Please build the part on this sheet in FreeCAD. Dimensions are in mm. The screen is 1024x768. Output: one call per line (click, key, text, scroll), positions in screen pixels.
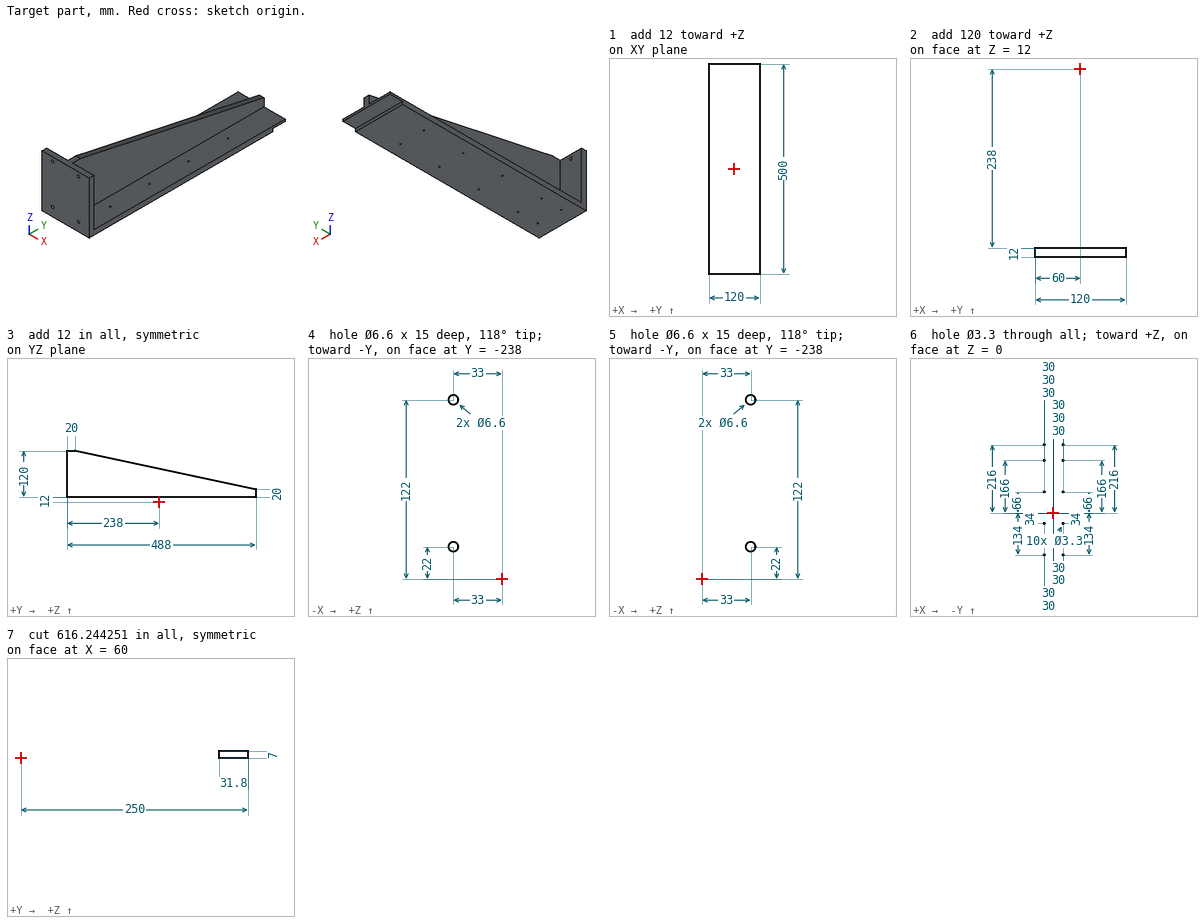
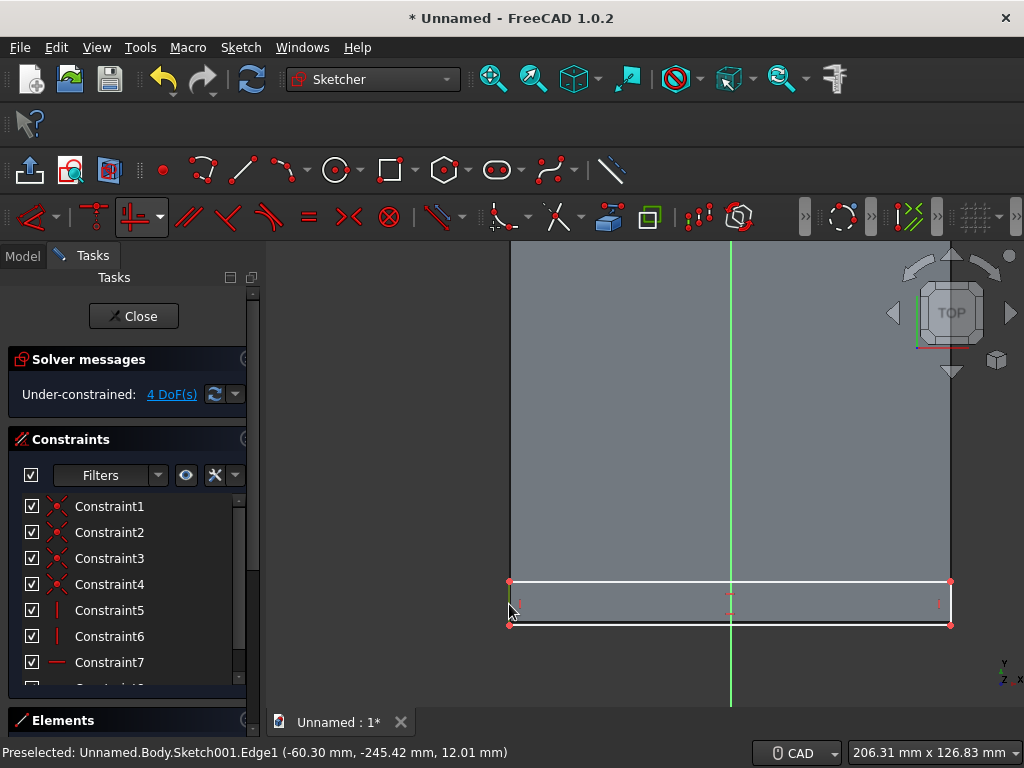
click(58, 218)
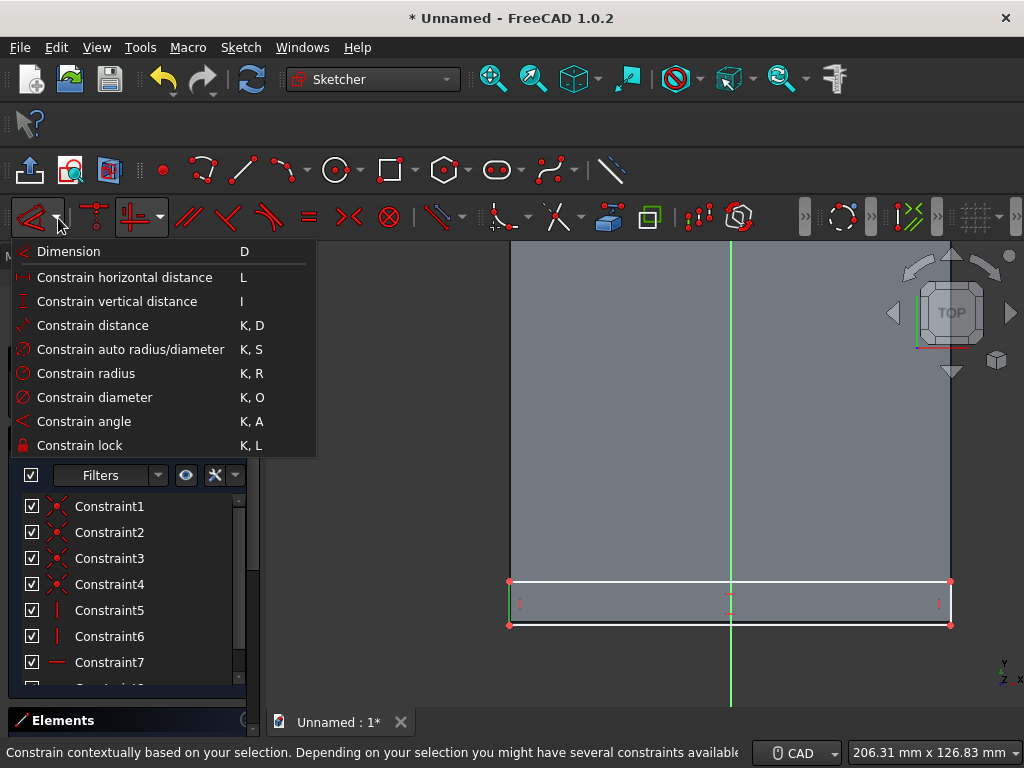
click(164, 301)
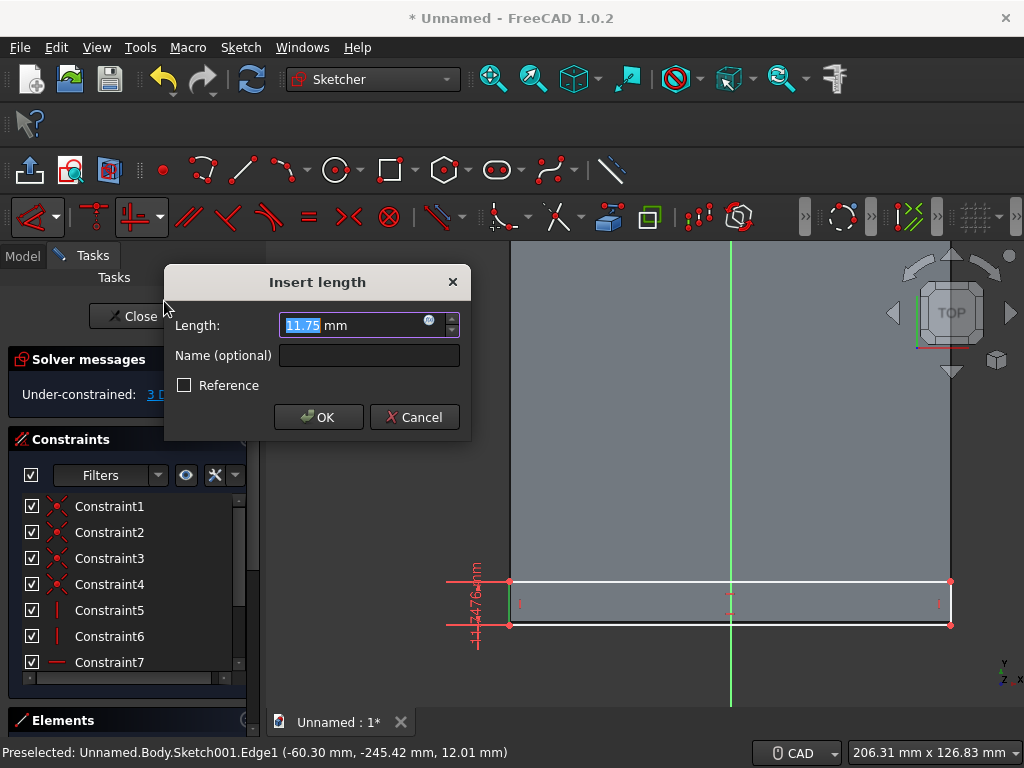
text(12)
key(Return)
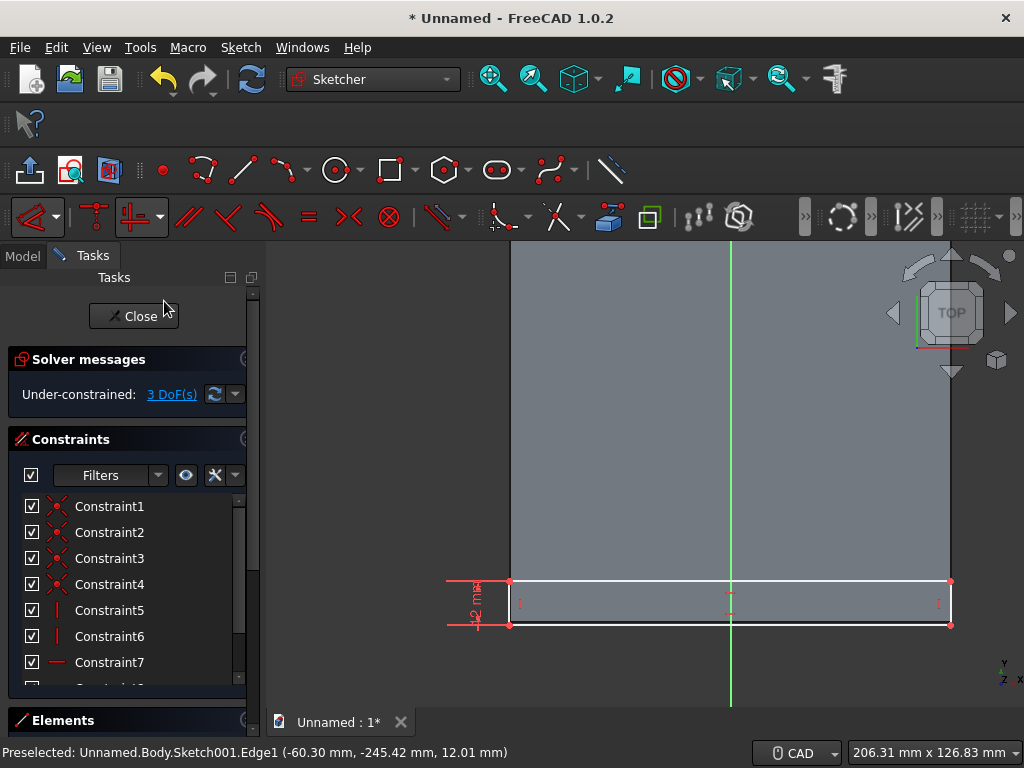
click(642, 625)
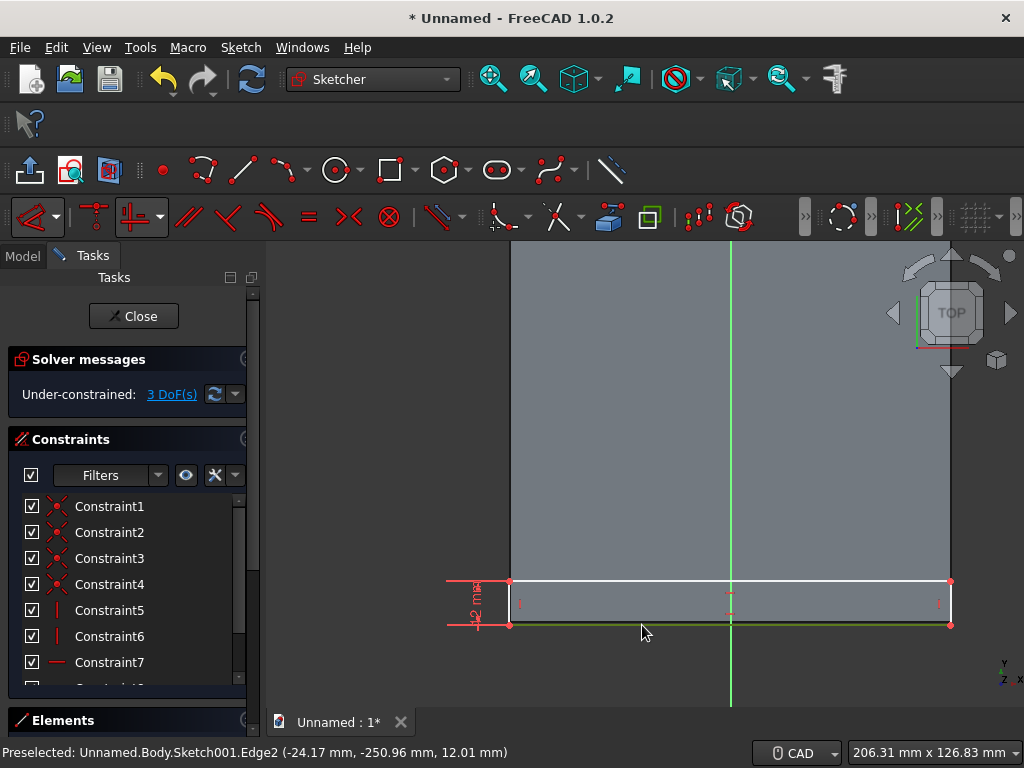
click(58, 218)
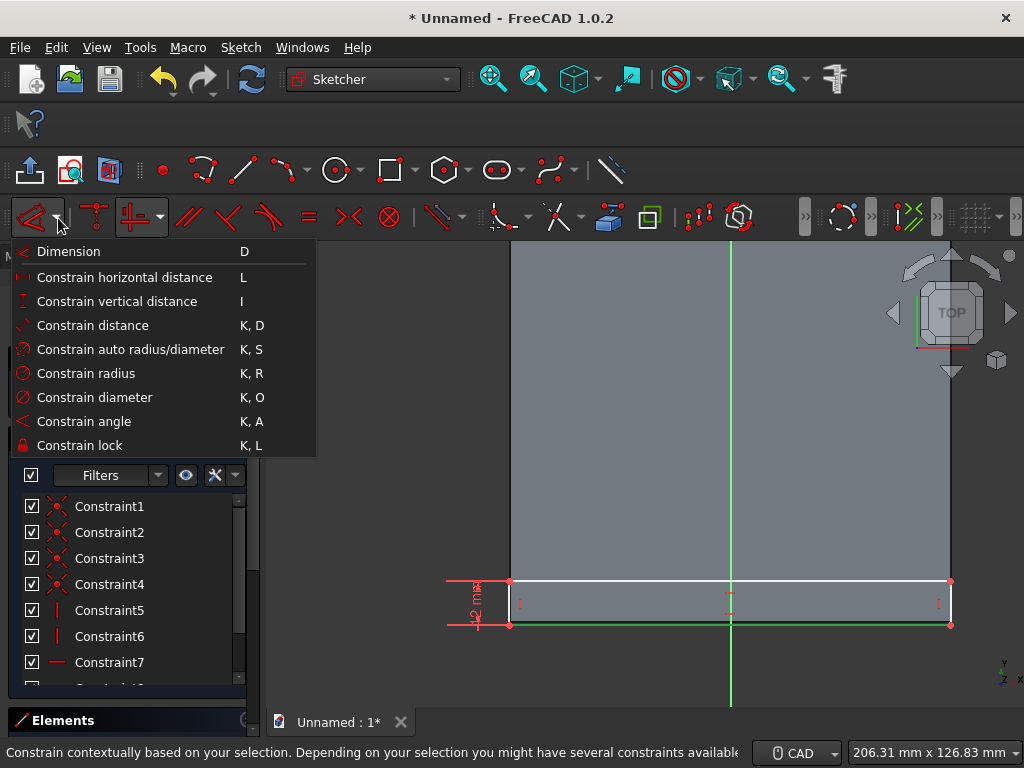
click(164, 277)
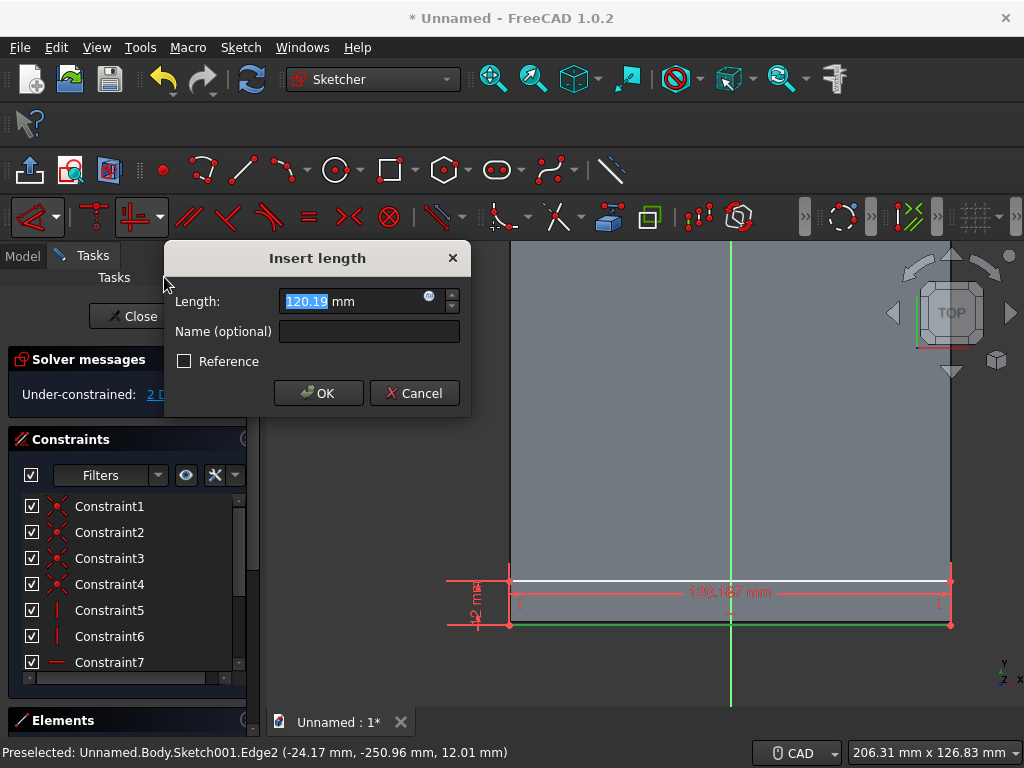
text(120)
key(Return)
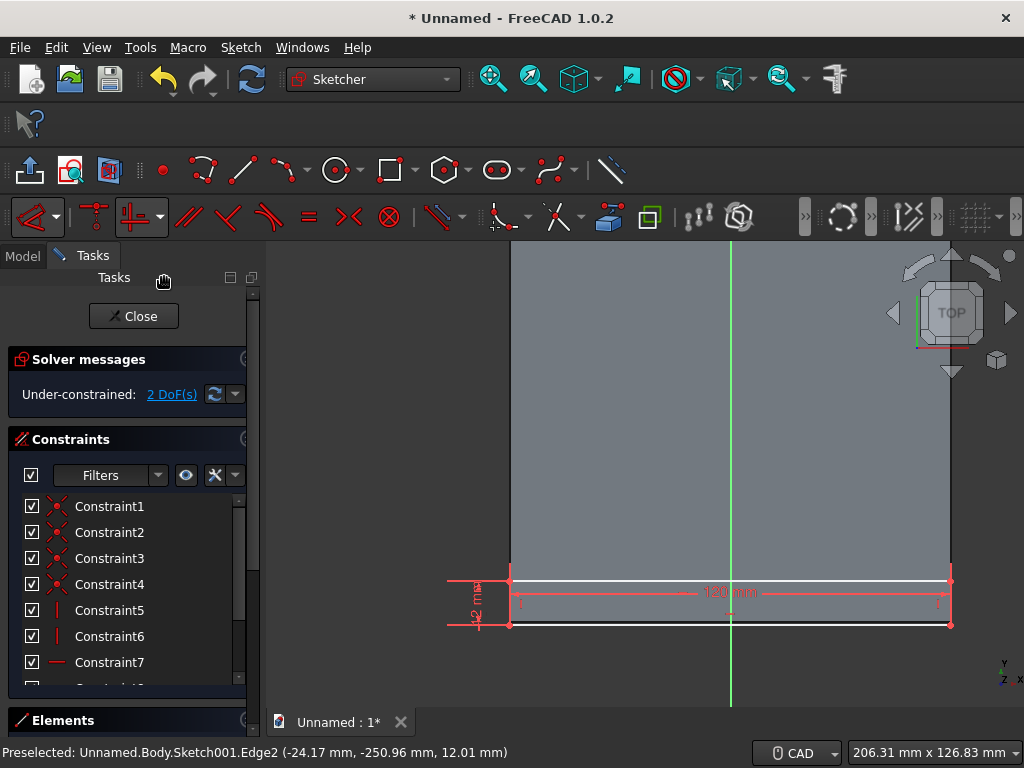
click(510, 581)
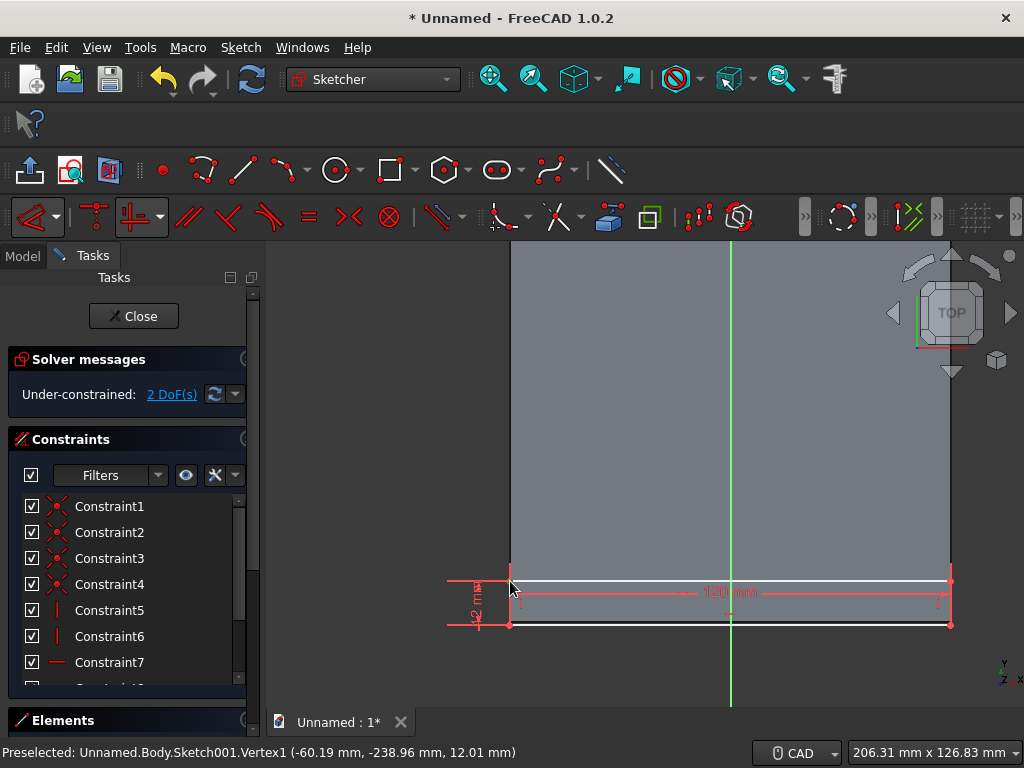
click(58, 218)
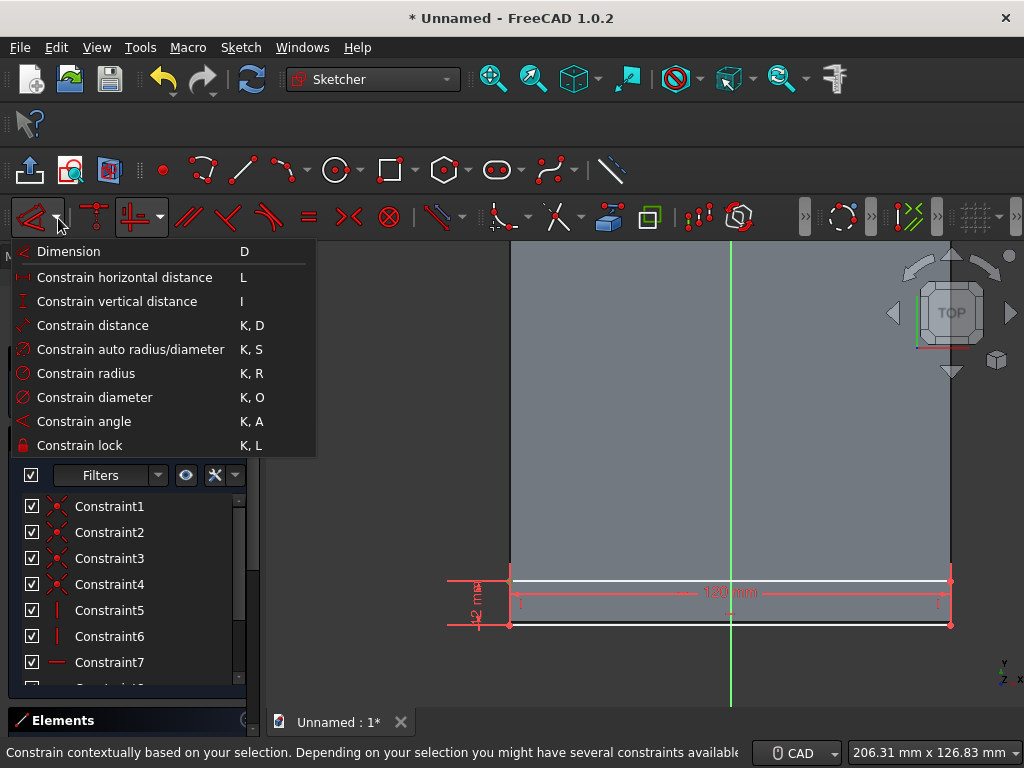
click(164, 277)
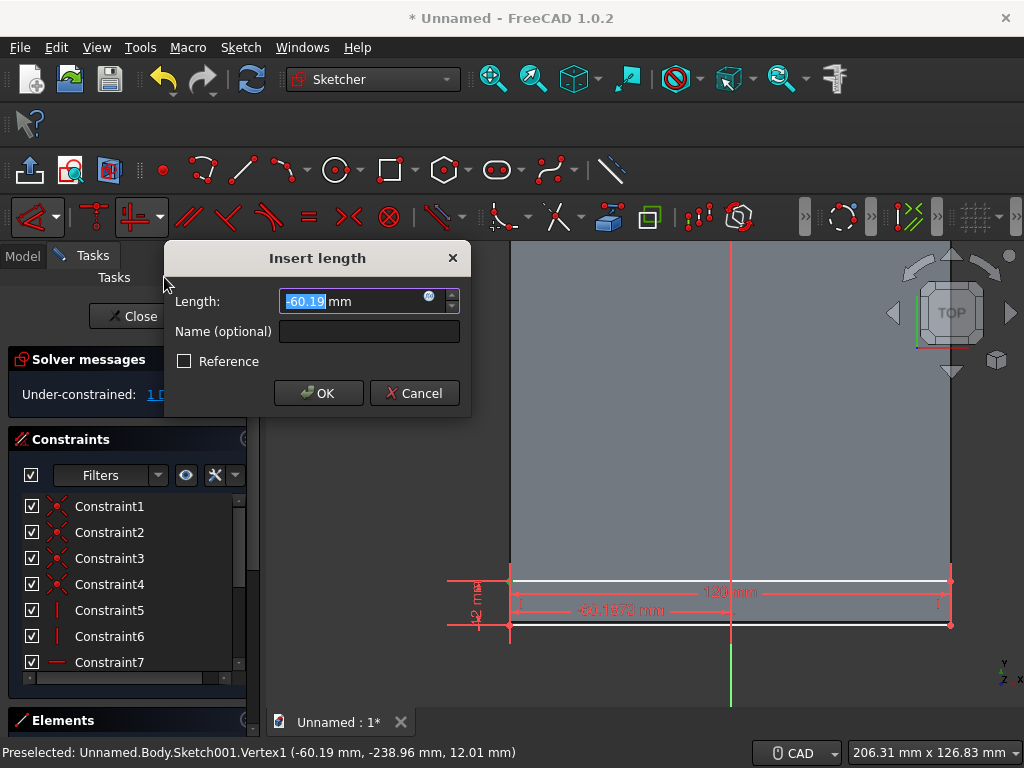
text(-60)
key(Return)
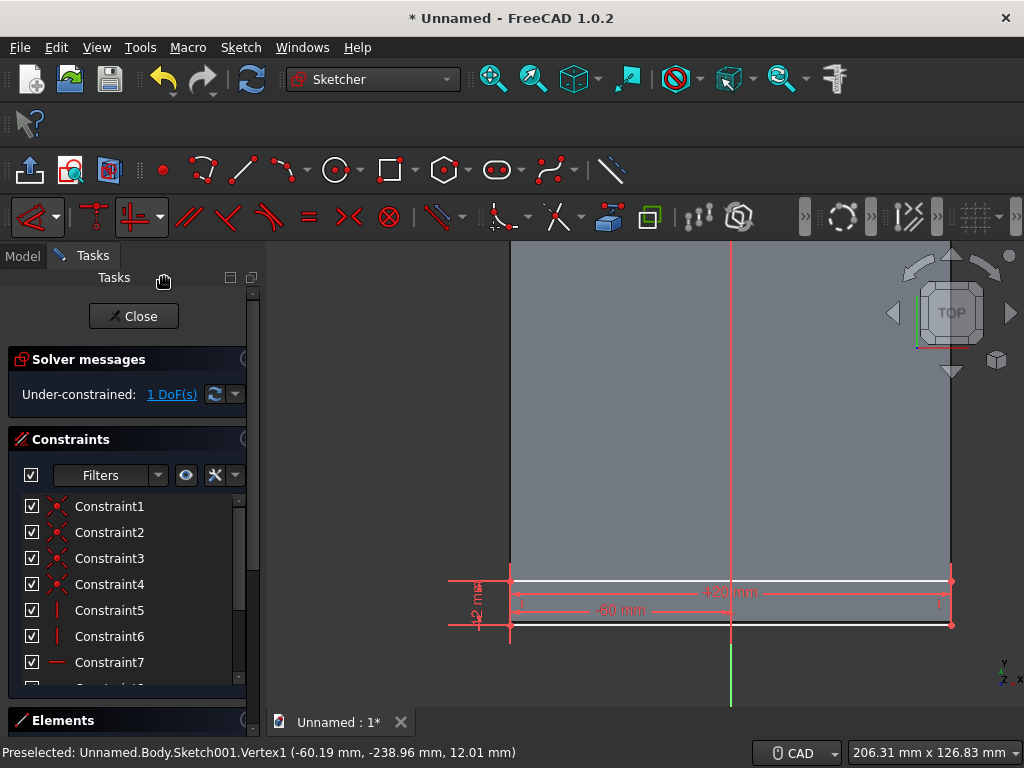
click(510, 581)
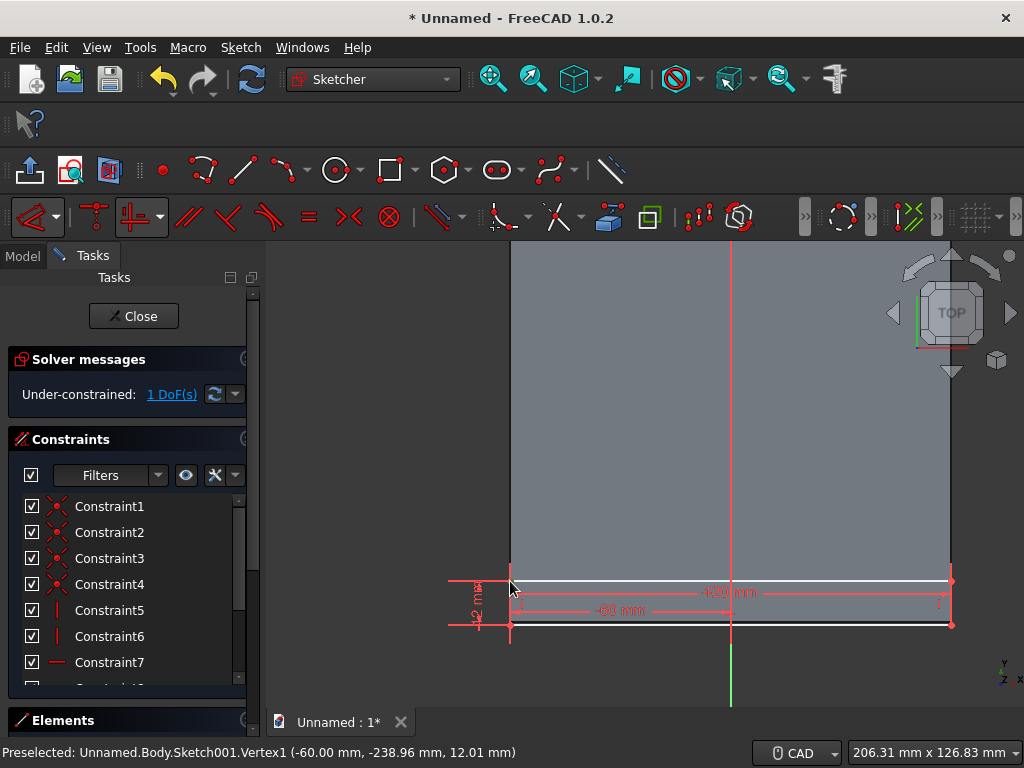
key(i)